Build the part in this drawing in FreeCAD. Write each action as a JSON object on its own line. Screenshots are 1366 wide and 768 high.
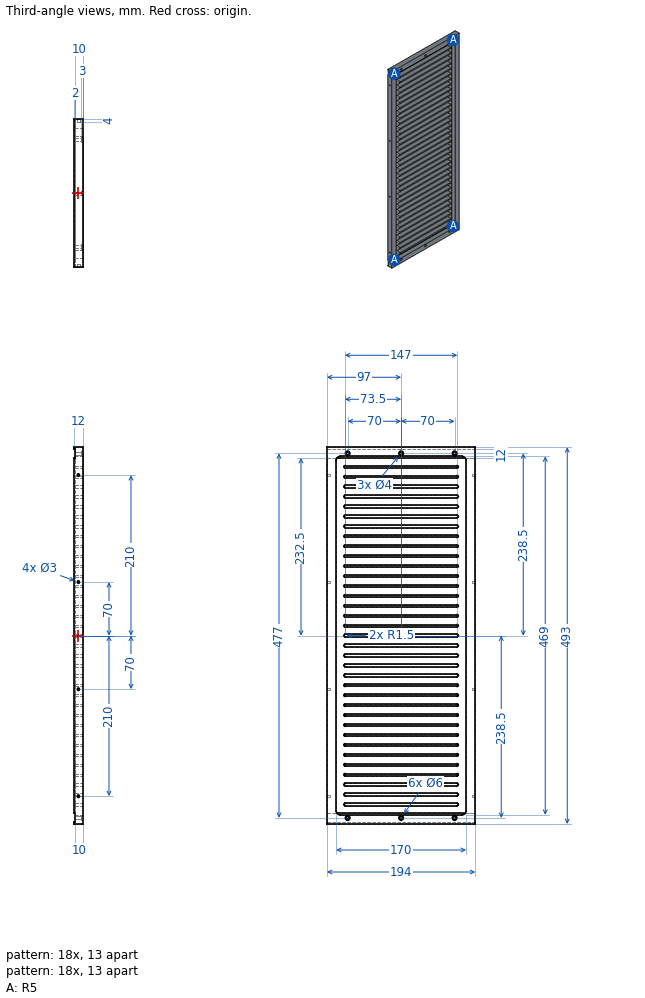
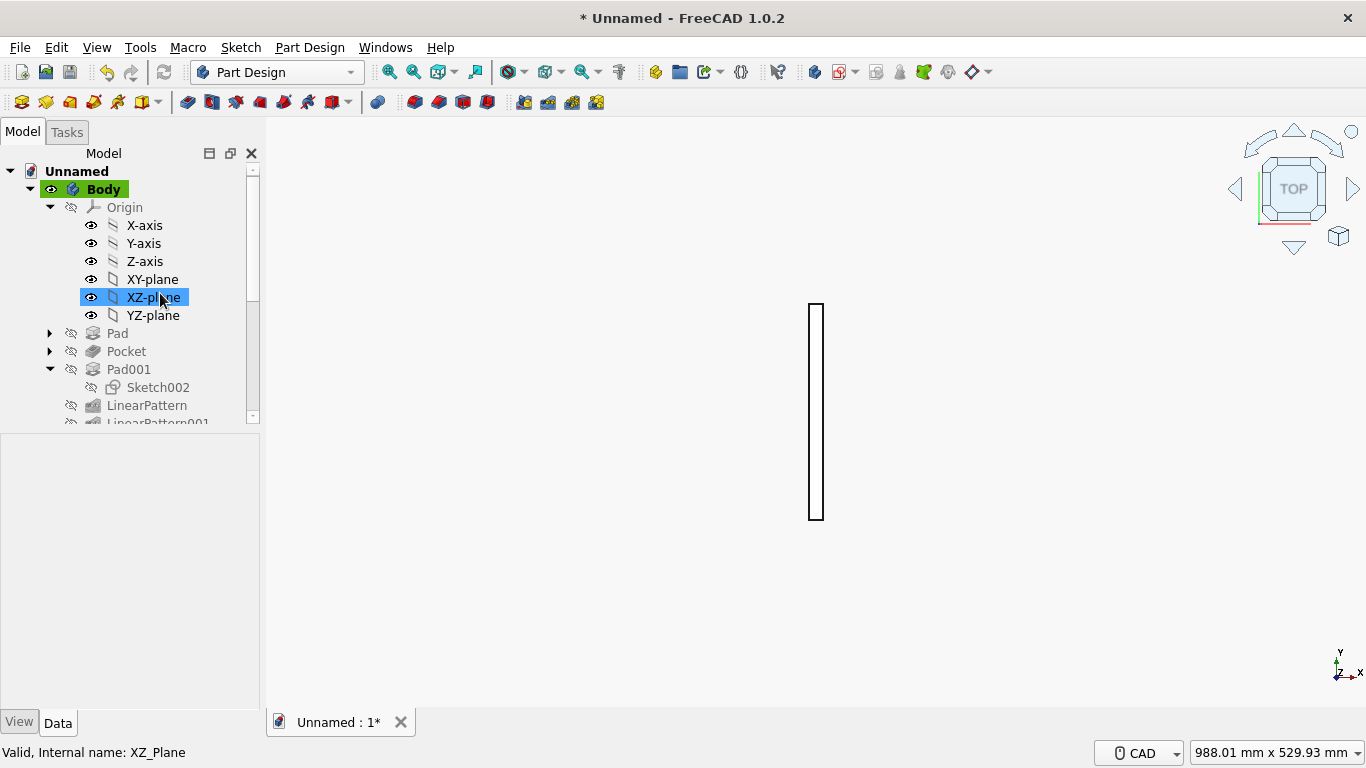
{"action": "left_click", "coordinate": [136, 315]}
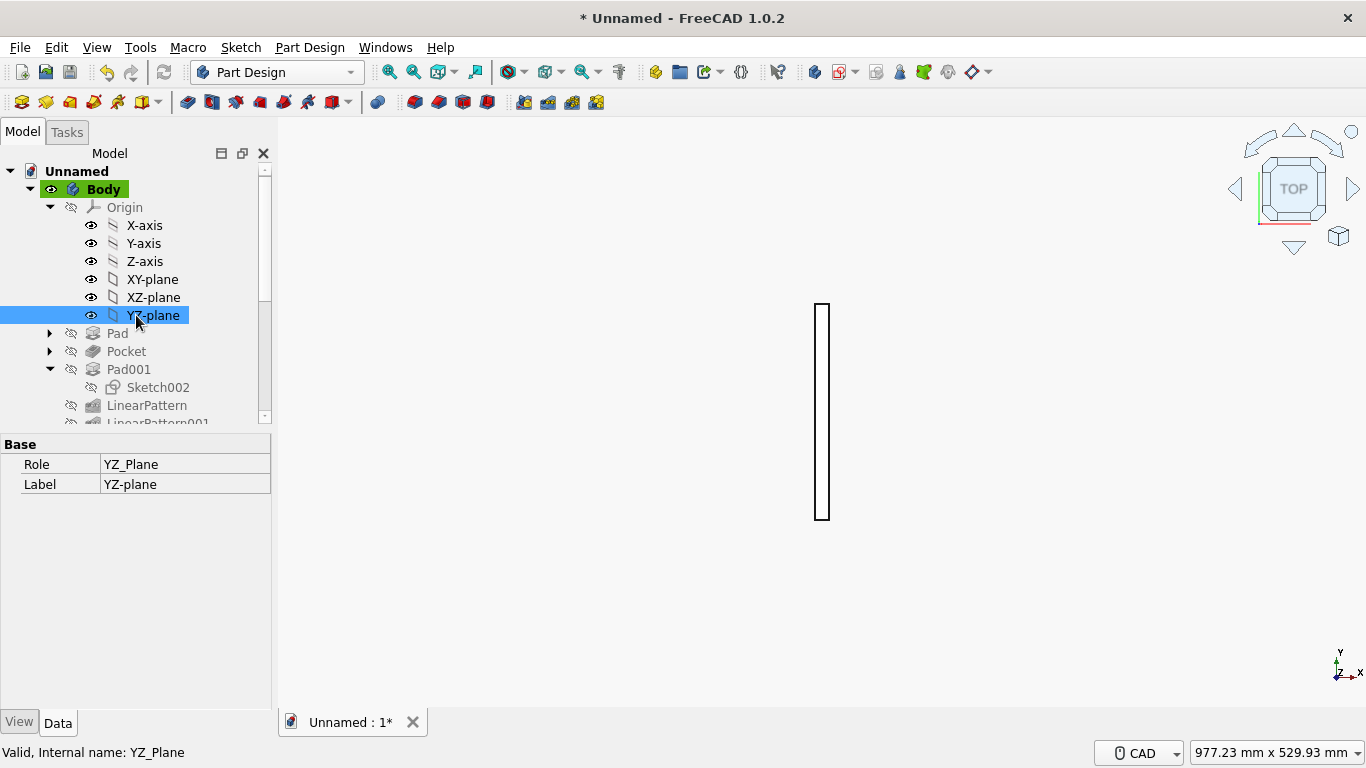
{"action": "left_click", "coordinate": [972, 72]}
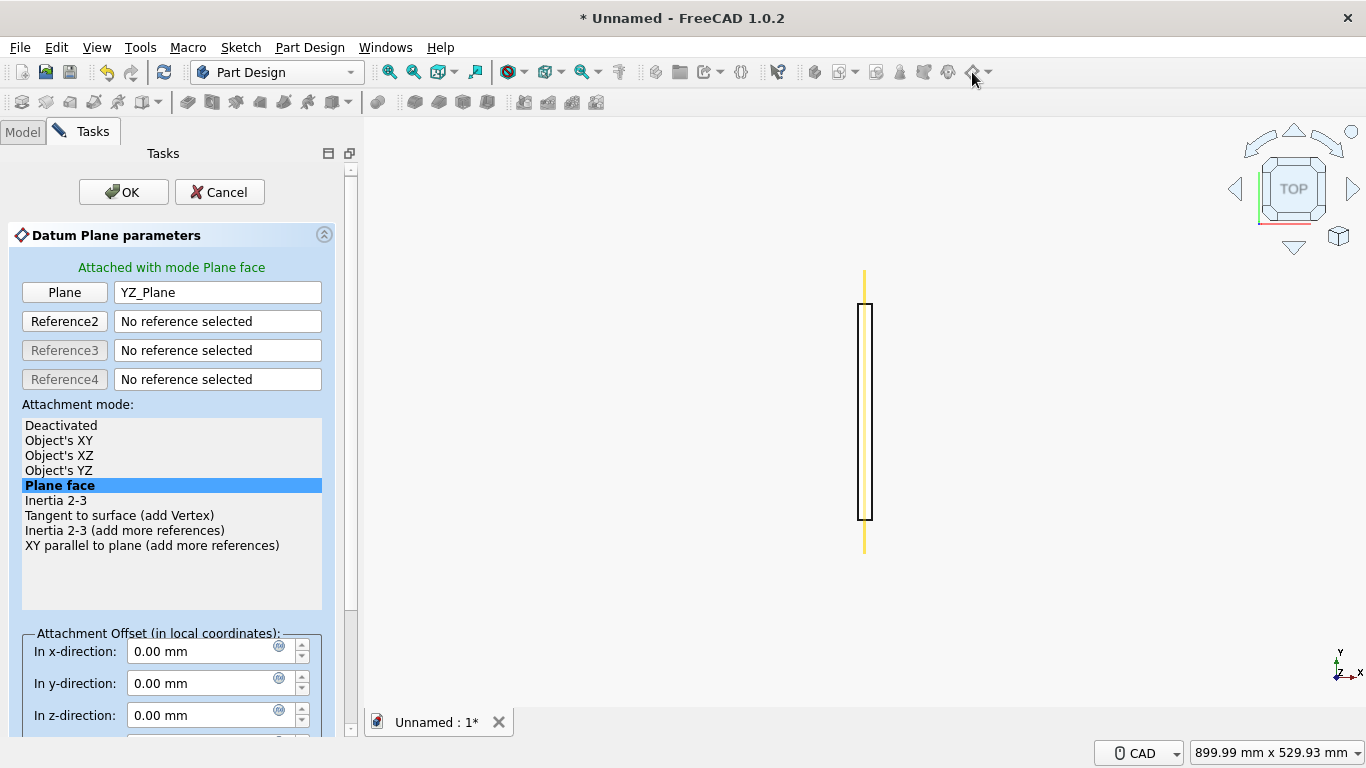
{"action": "triple_click", "coordinate": [210, 715]}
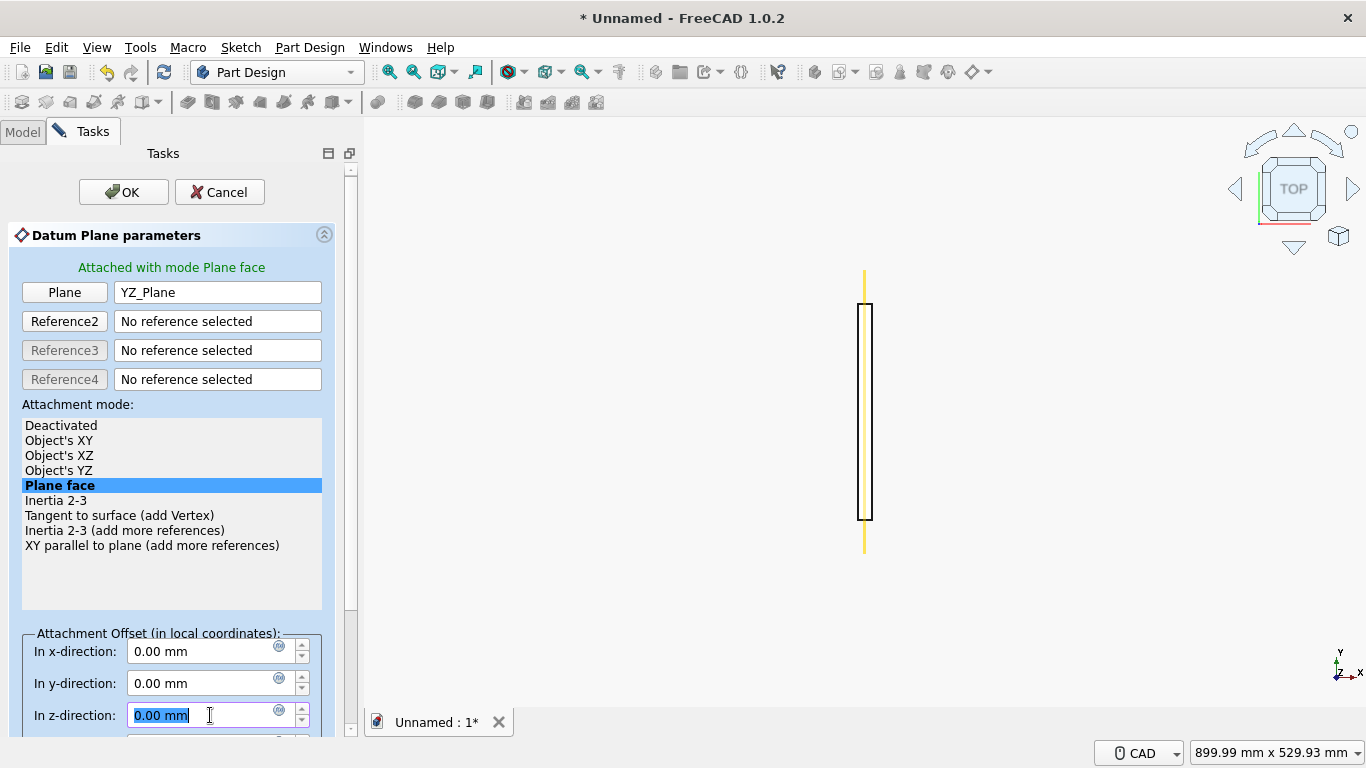
{"action": "type", "text": "6"}
{"action": "key", "text": "Tab"}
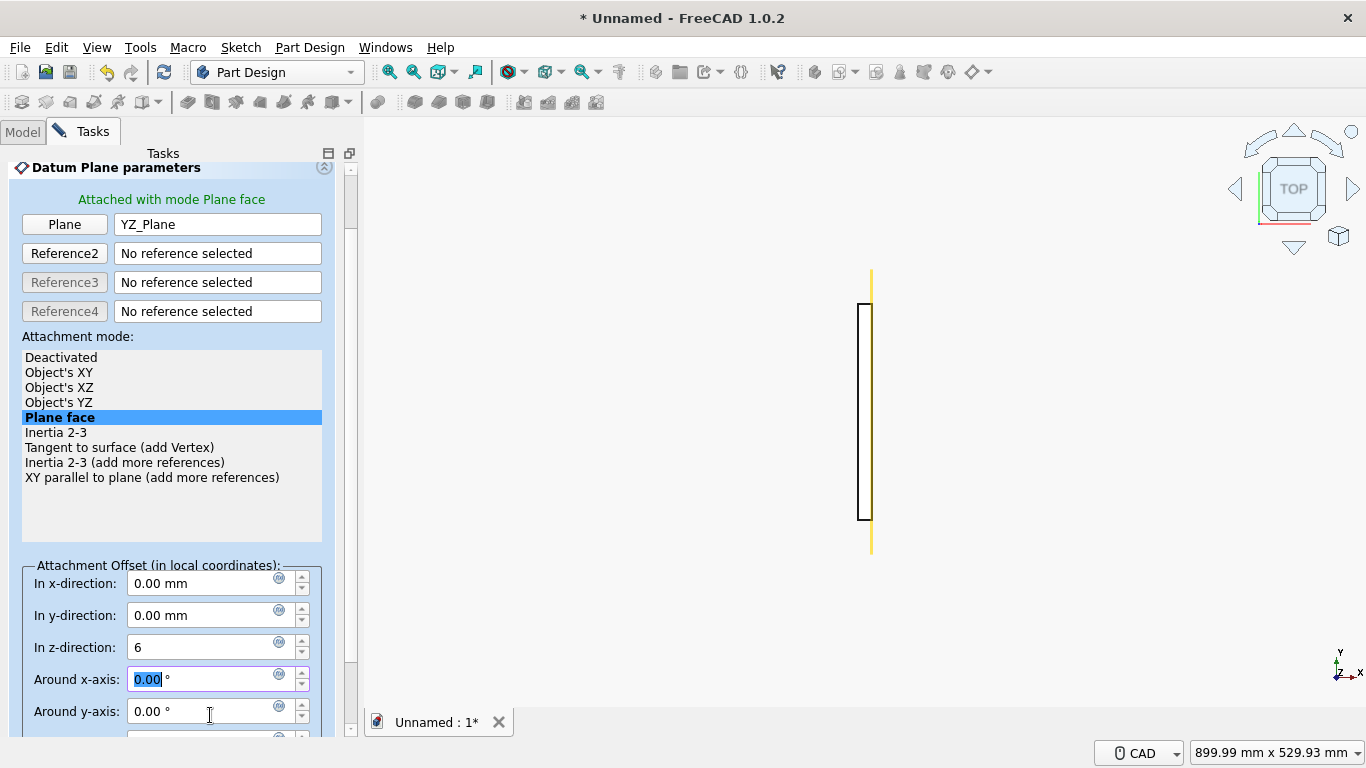
{"action": "scroll", "coordinate": [351, 450], "scroll_direction": "up", "scroll_amount": 2}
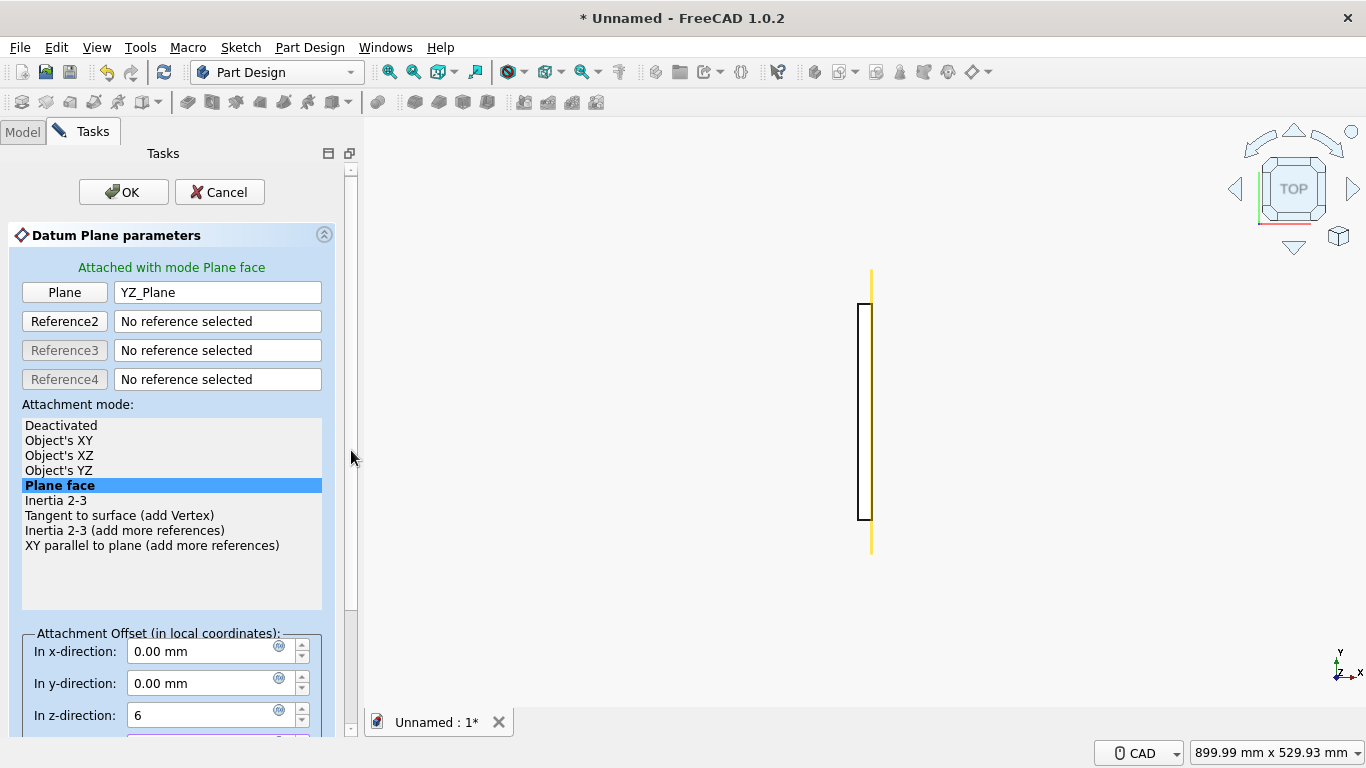
{"action": "left_click", "coordinate": [124, 192]}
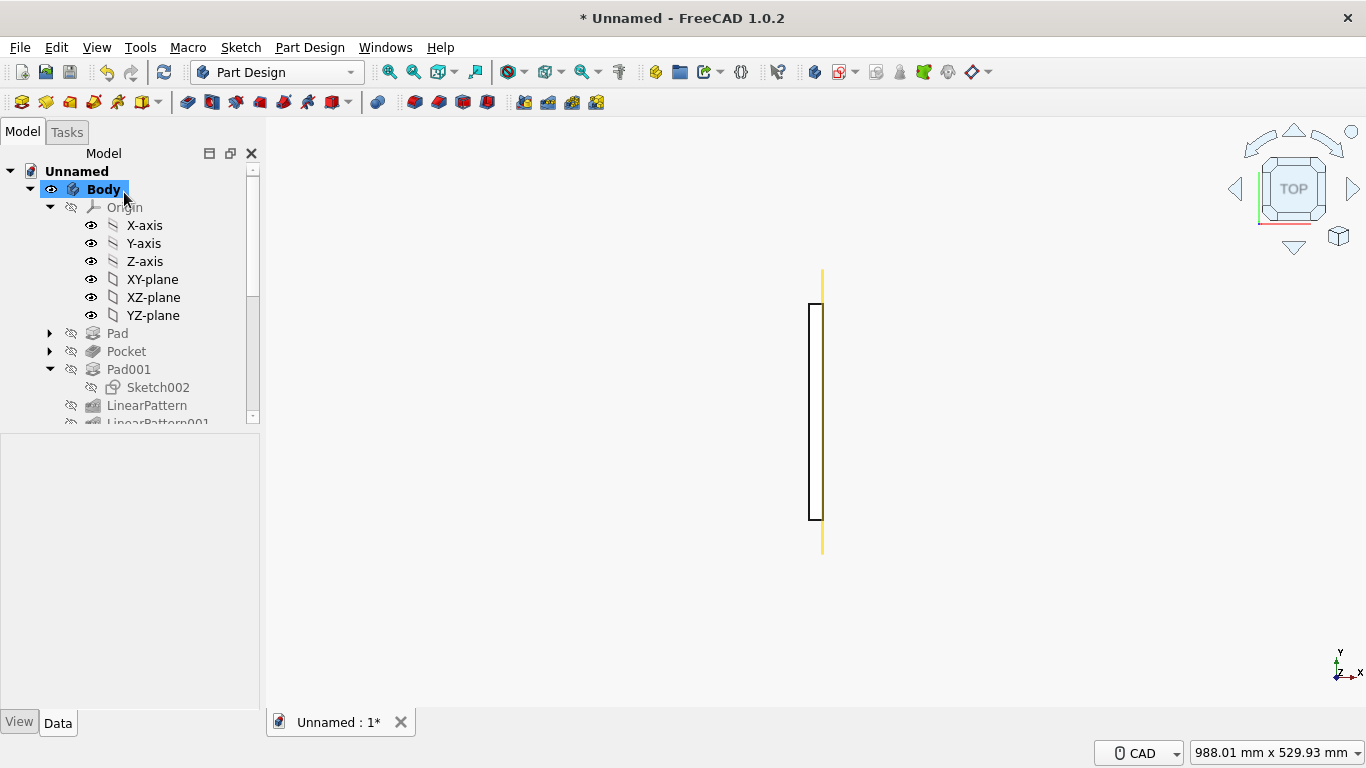
{"action": "scroll", "coordinate": [100, 293], "scroll_direction": "down", "scroll_amount": 3}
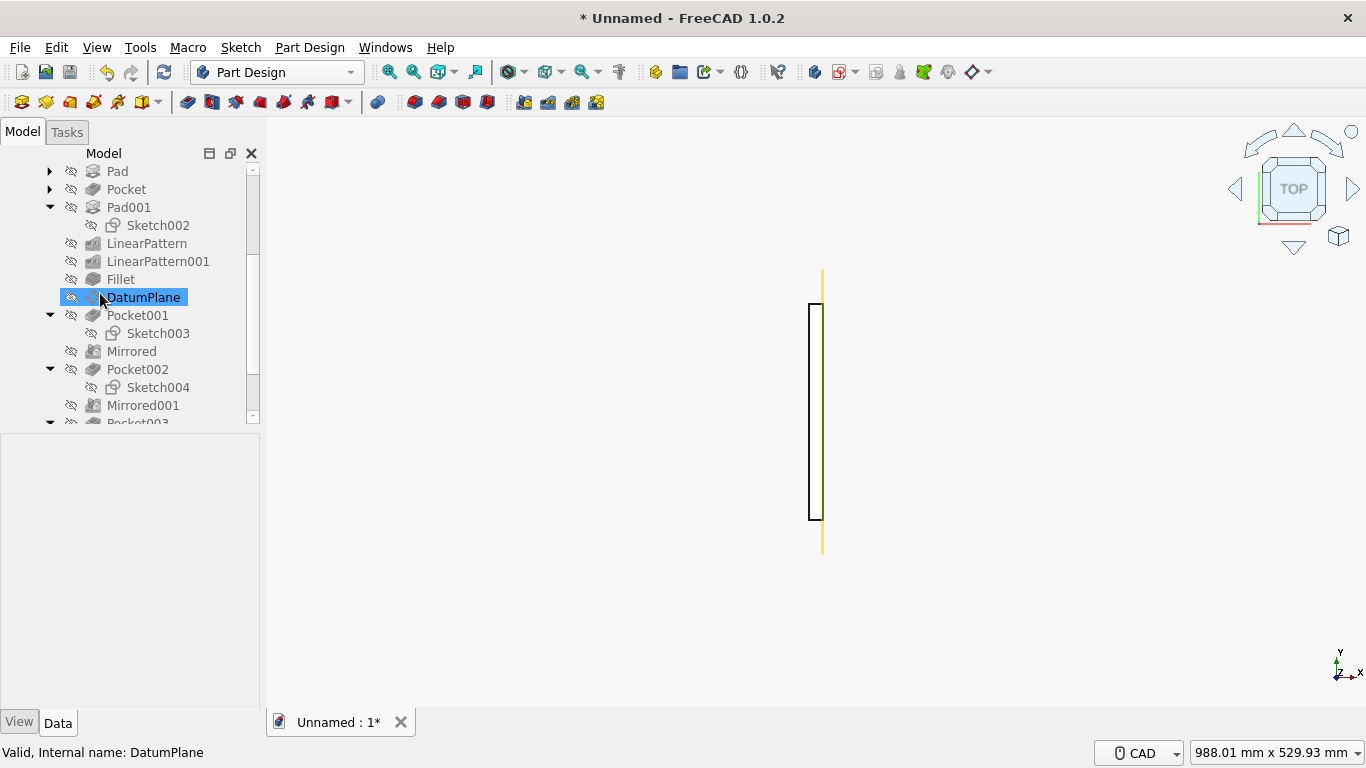
{"action": "scroll", "coordinate": [140, 293], "scroll_direction": "up", "scroll_amount": 15}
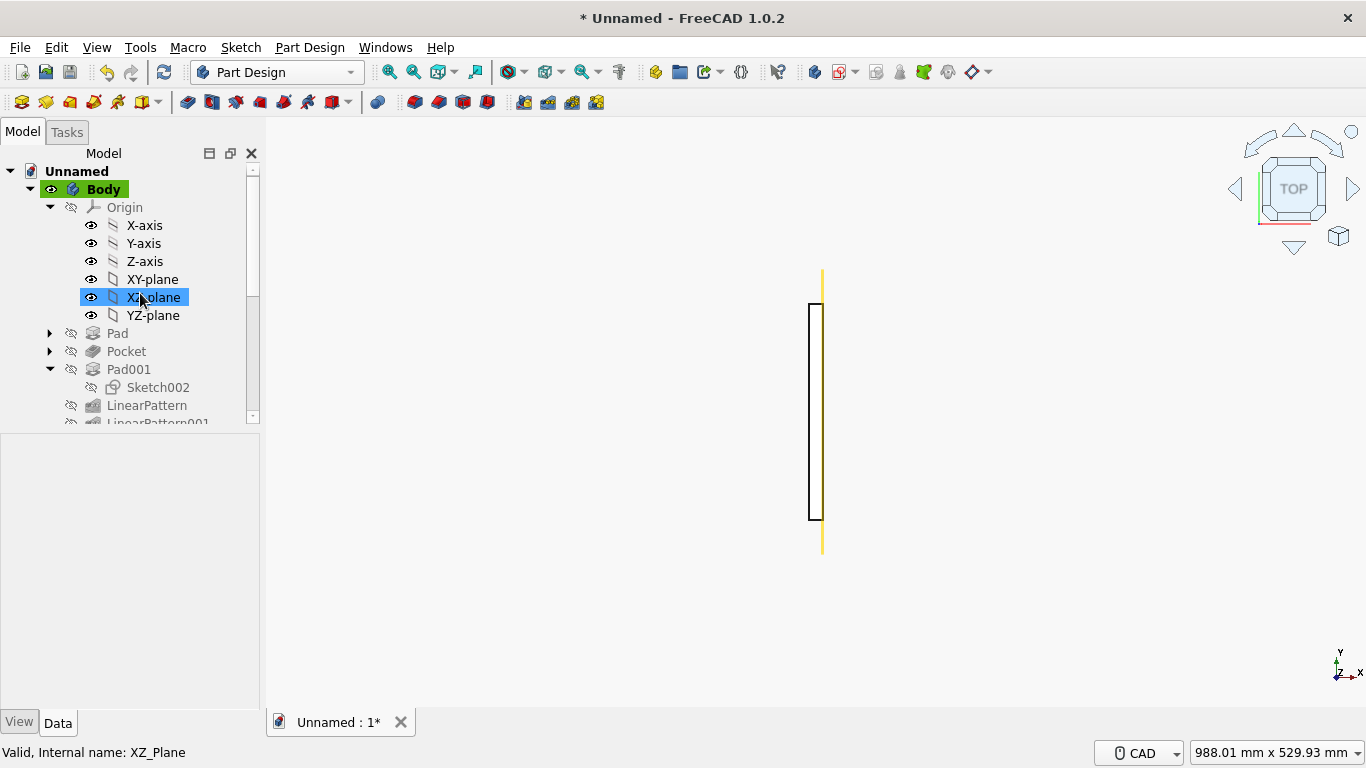
{"action": "scroll", "coordinate": [100, 293], "scroll_direction": "down", "scroll_amount": 6}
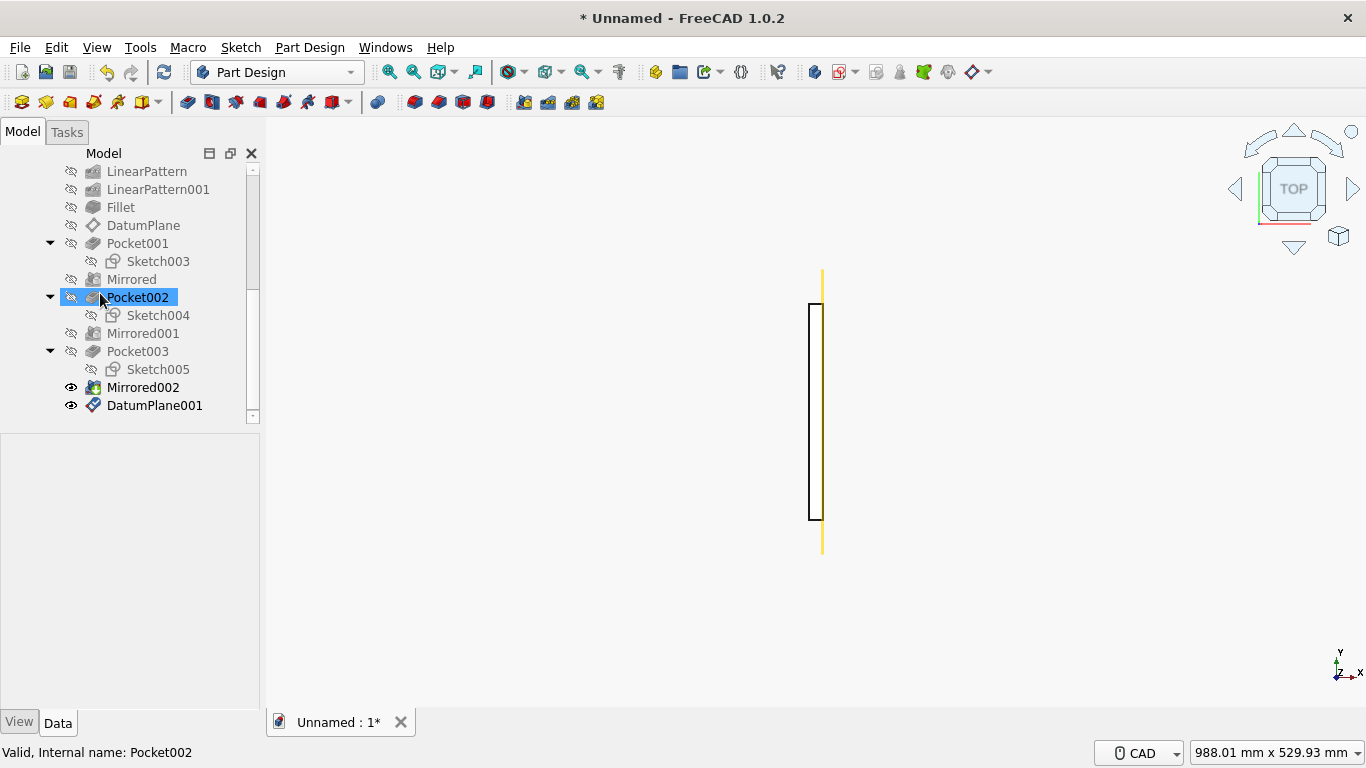
{"action": "left_click", "coordinate": [116, 405]}